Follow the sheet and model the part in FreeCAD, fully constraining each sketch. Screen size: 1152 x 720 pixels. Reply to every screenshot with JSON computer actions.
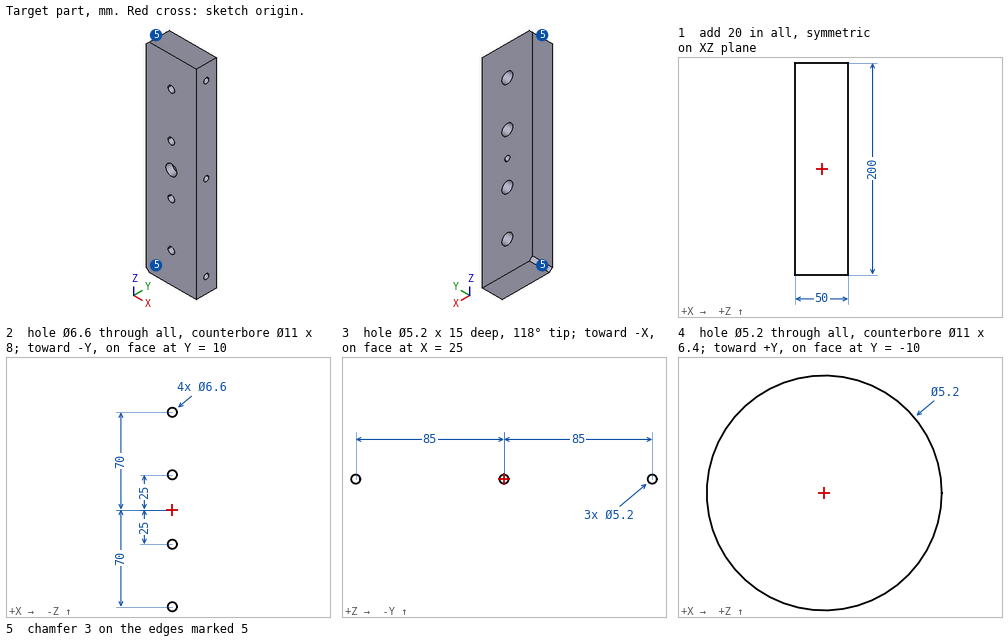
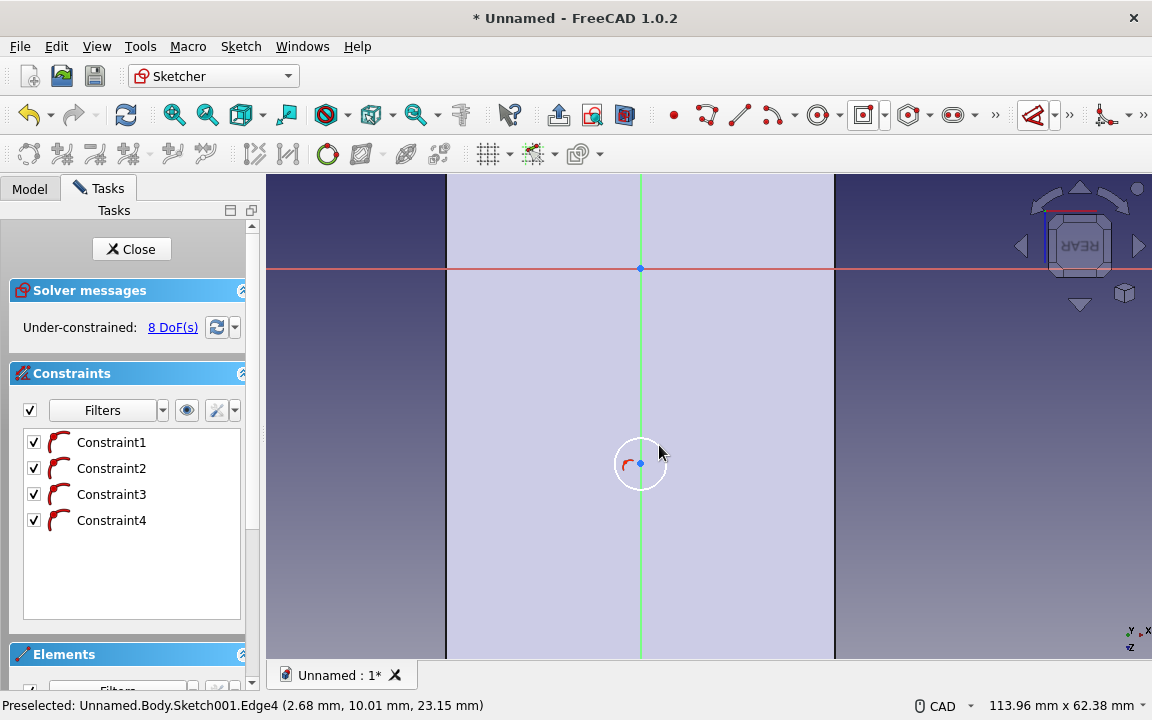
{"action": "scroll", "coordinate": [640, 465], "scroll_direction": "down", "scroll_amount": 7}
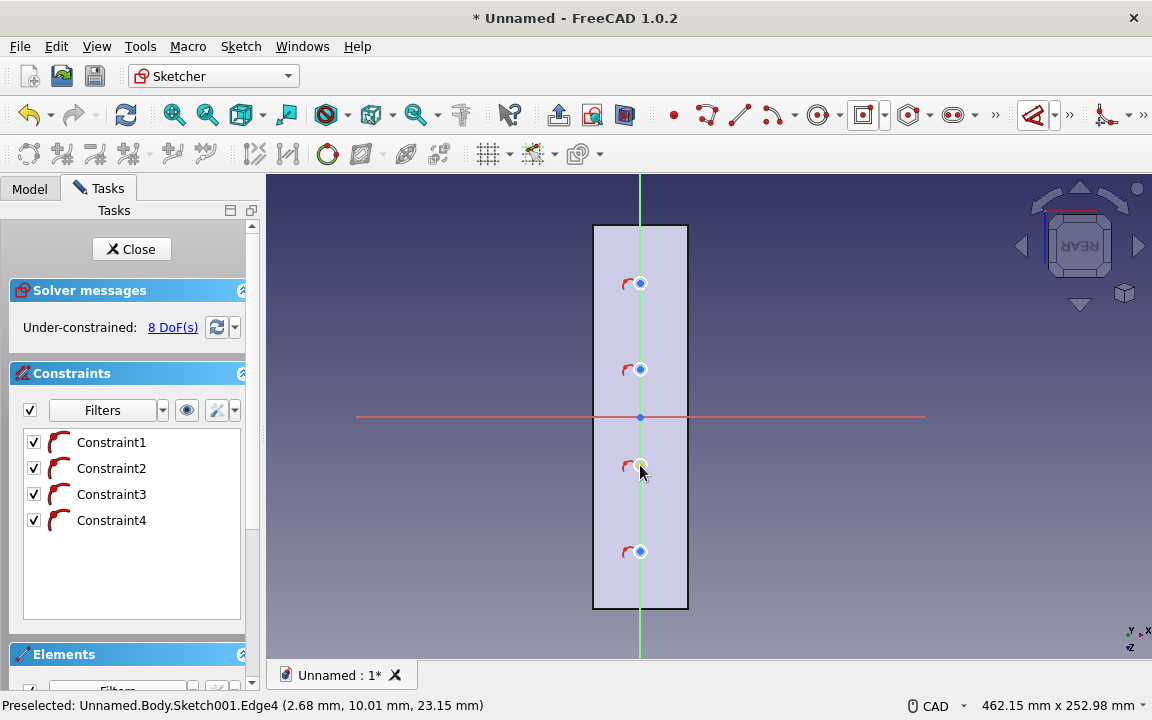
{"action": "scroll", "coordinate": [645, 279], "scroll_direction": "up", "scroll_amount": 6}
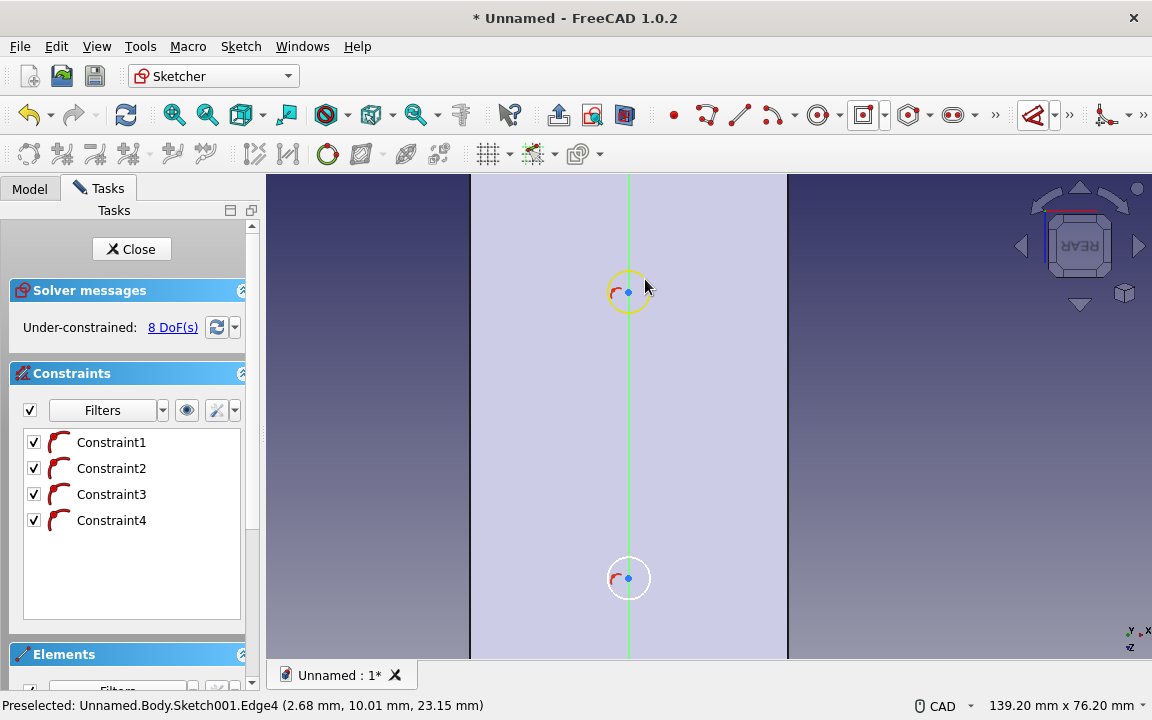
{"action": "left_click", "coordinate": [644, 277]}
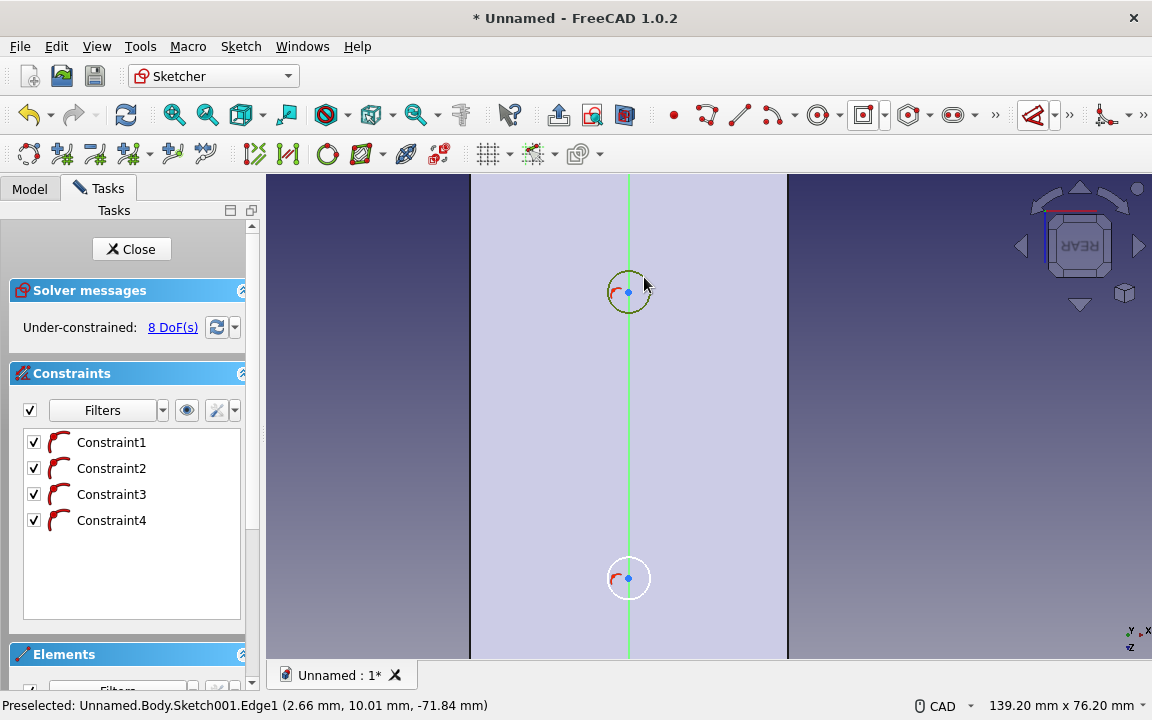
{"action": "scroll", "coordinate": [645, 278], "scroll_direction": "down", "scroll_amount": 6}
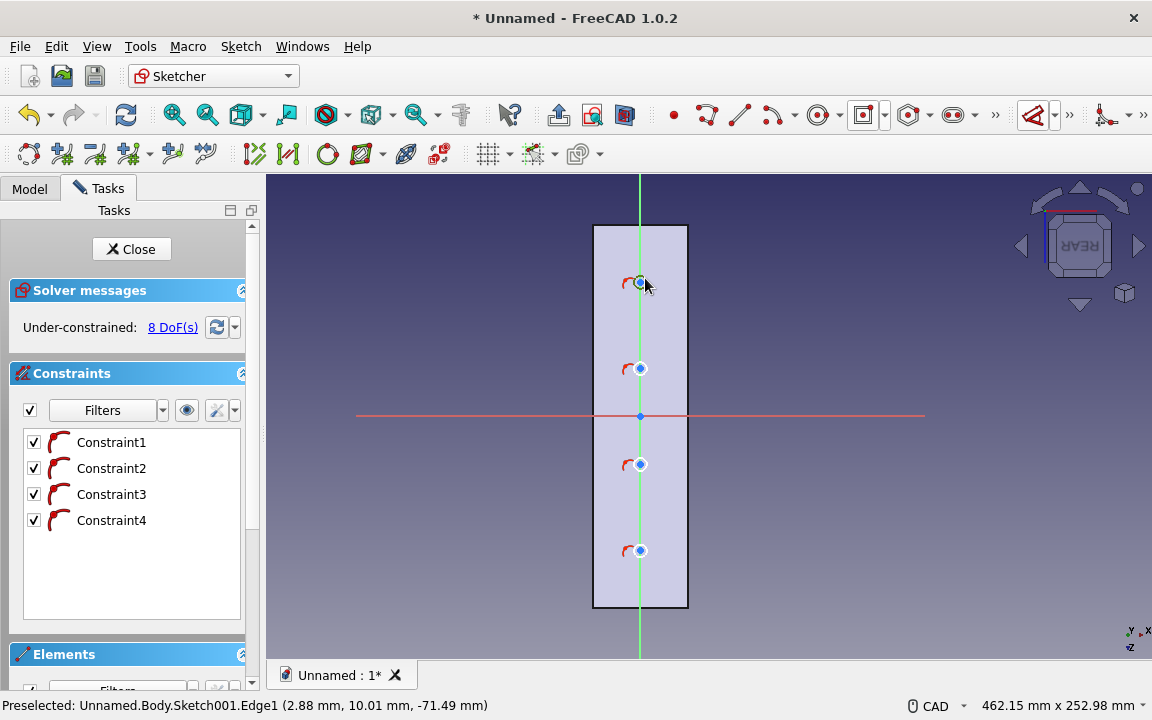
{"action": "scroll", "coordinate": [645, 546], "scroll_direction": "up", "scroll_amount": 6}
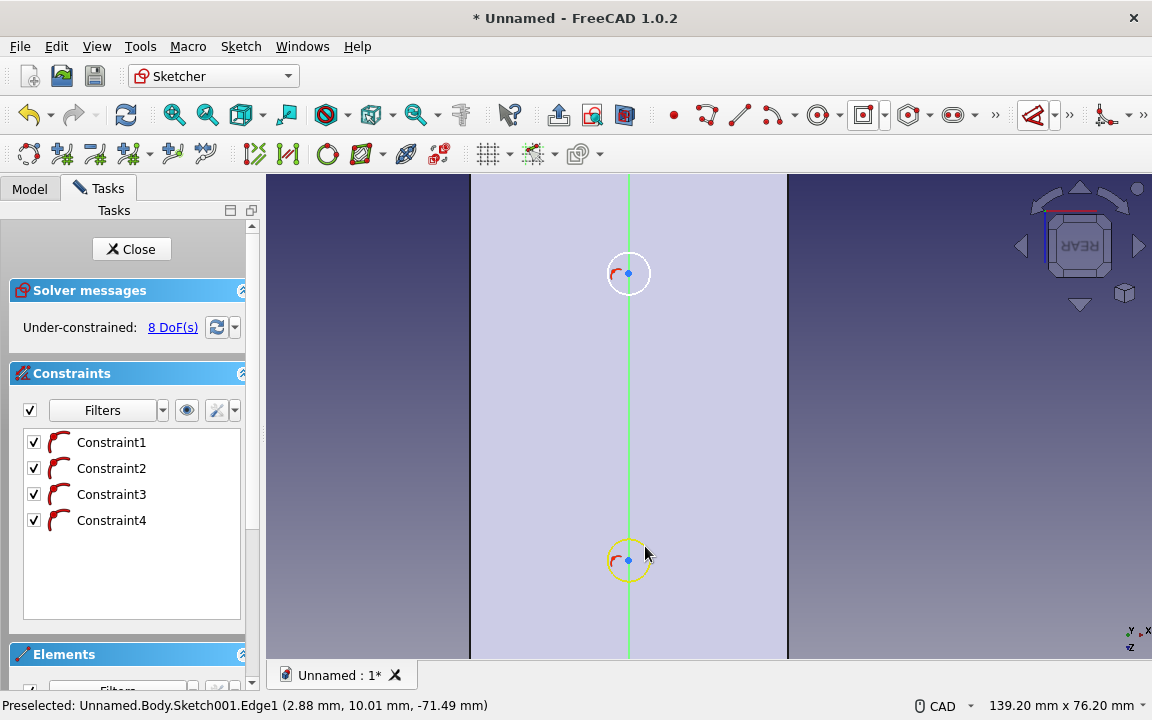
{"action": "left_click", "coordinate": [644, 546]}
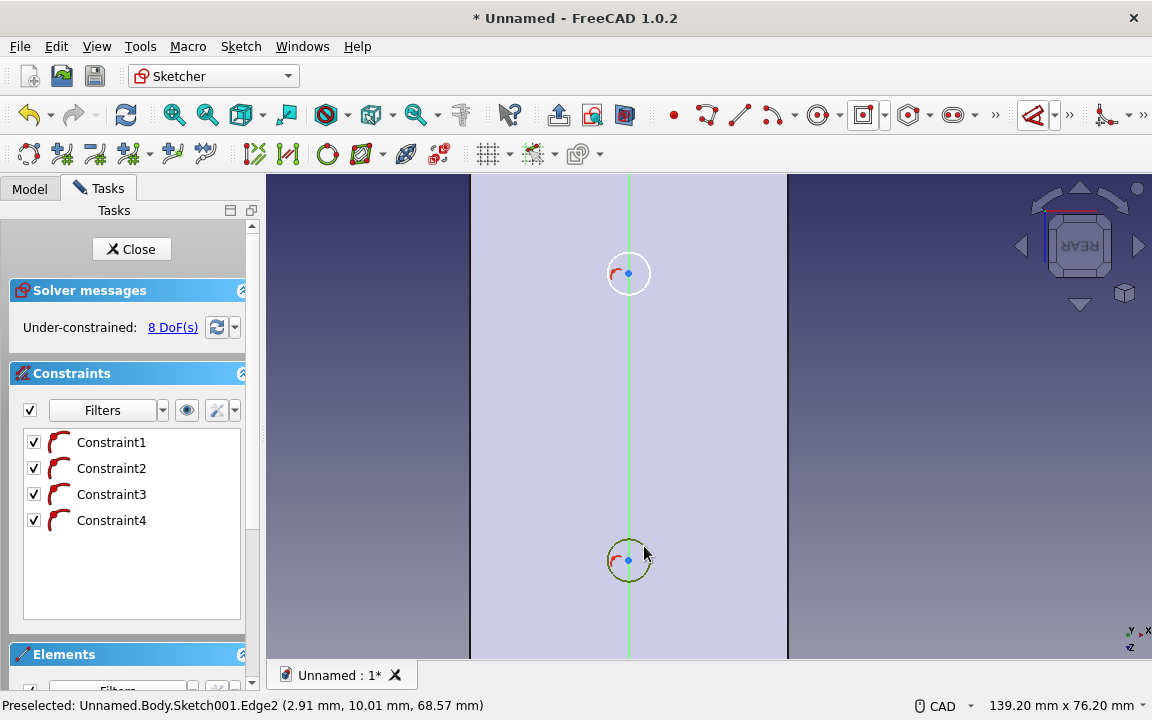
{"action": "scroll", "coordinate": [645, 547], "scroll_direction": "down", "scroll_amount": 6}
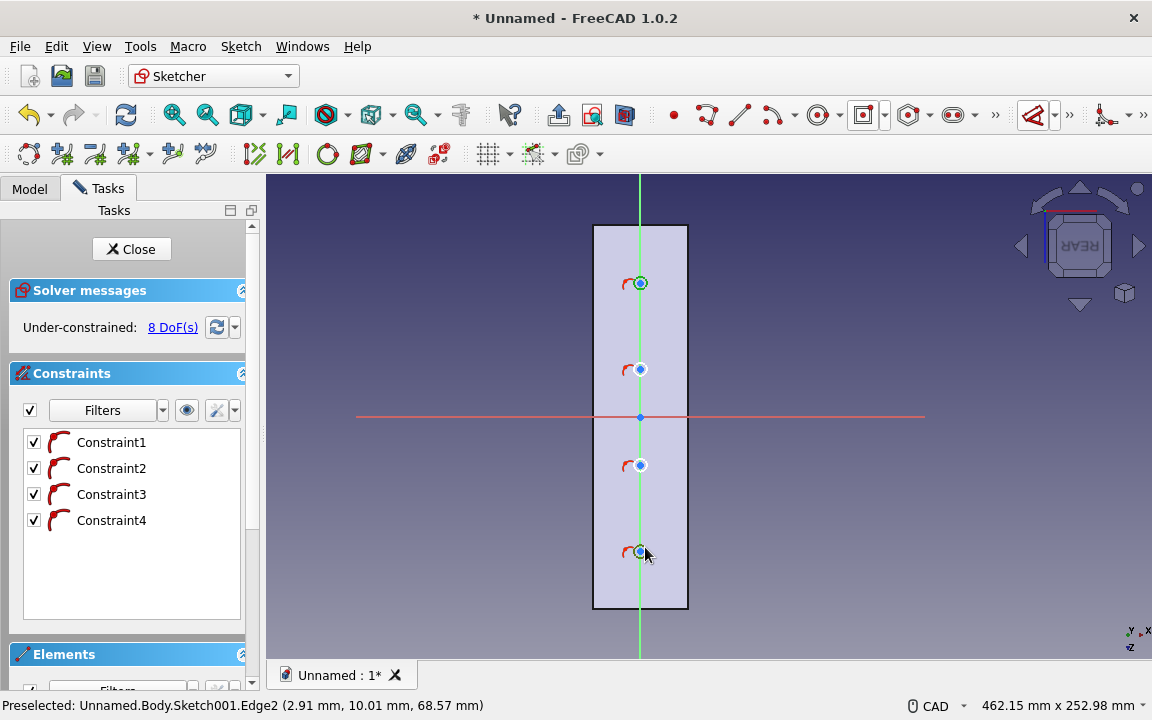
{"action": "scroll", "coordinate": [645, 365], "scroll_direction": "up", "scroll_amount": 6}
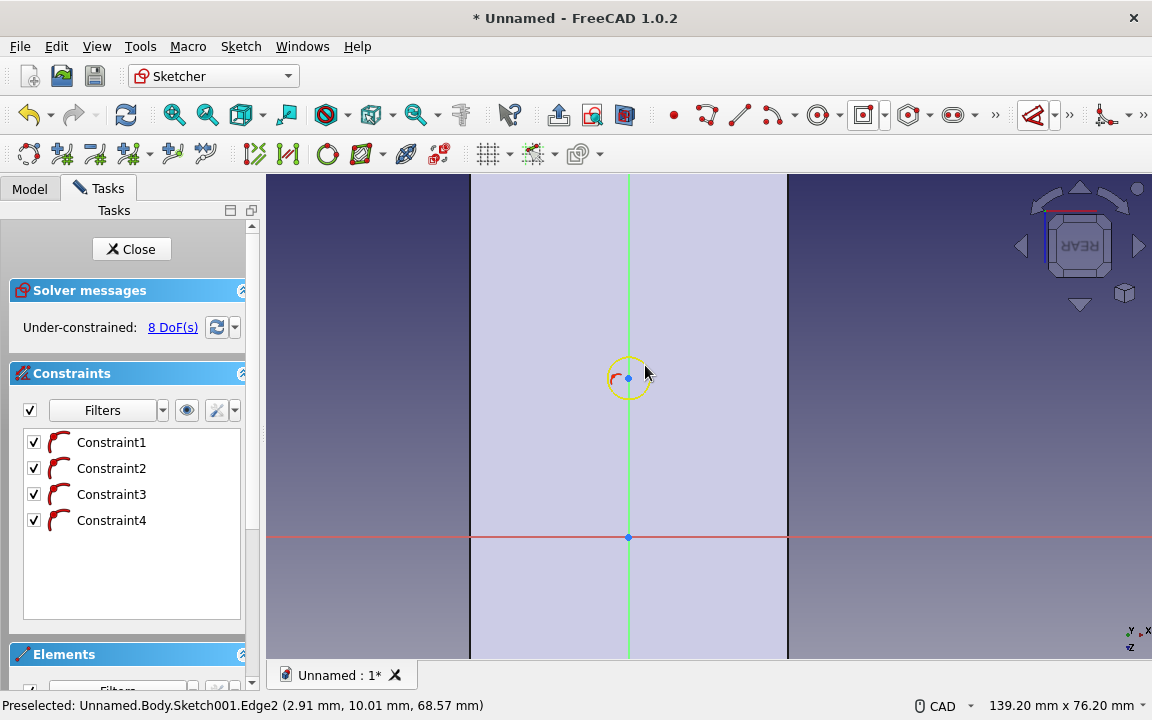
{"action": "left_click", "coordinate": [644, 363]}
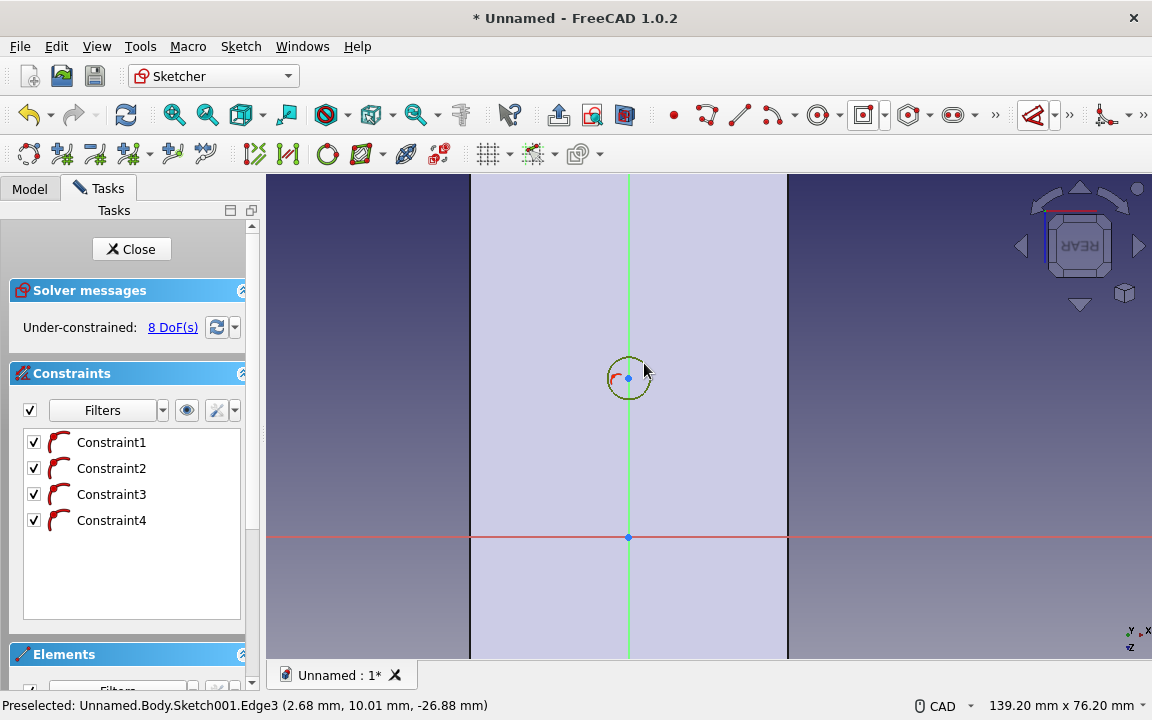
{"action": "scroll", "coordinate": [645, 365], "scroll_direction": "down", "scroll_amount": 6}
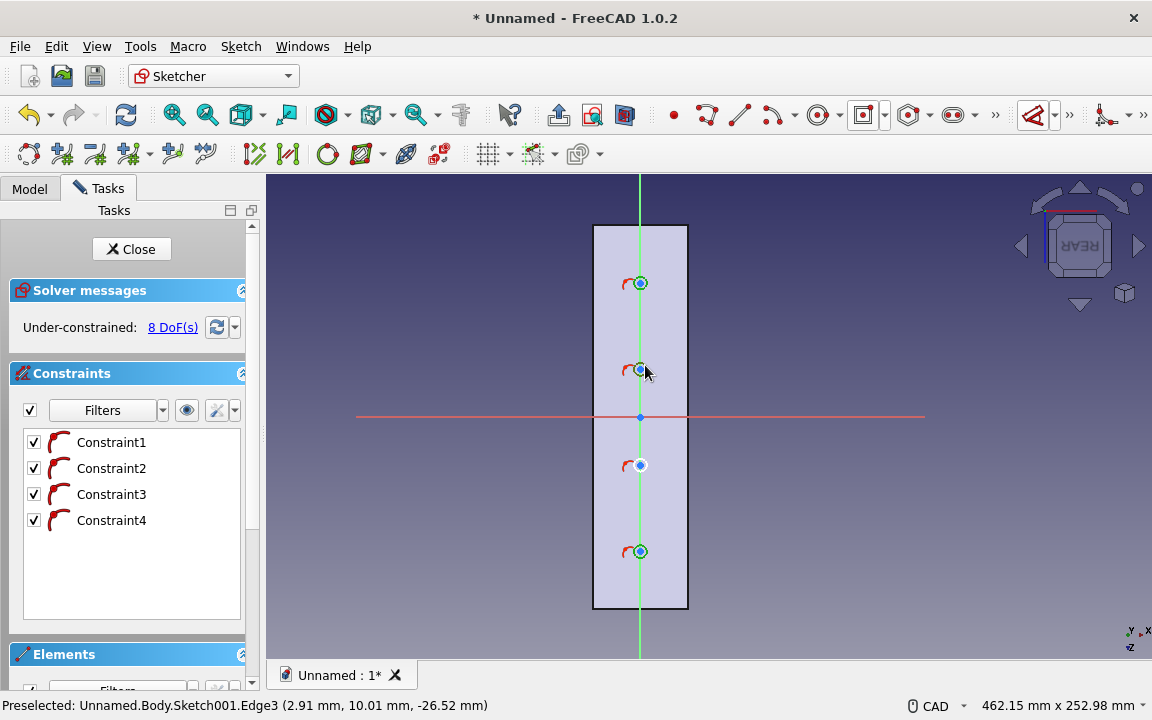
{"action": "scroll", "coordinate": [645, 461], "scroll_direction": "up", "scroll_amount": 6}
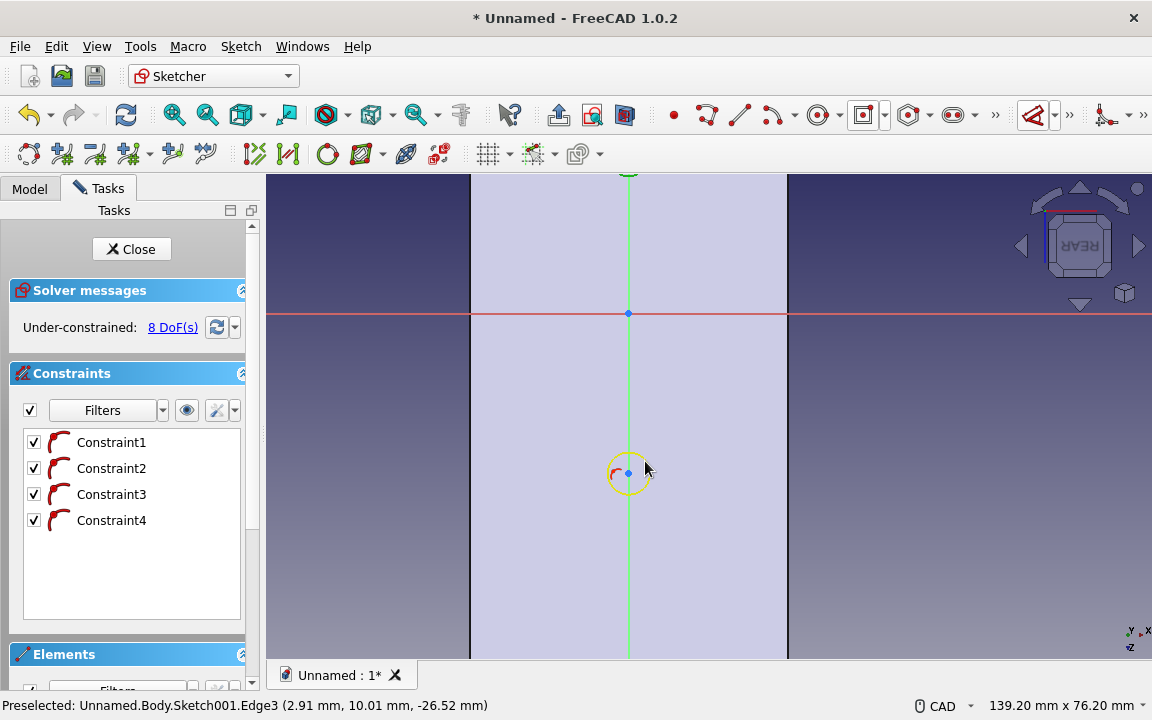
{"action": "left_click", "coordinate": [644, 459]}